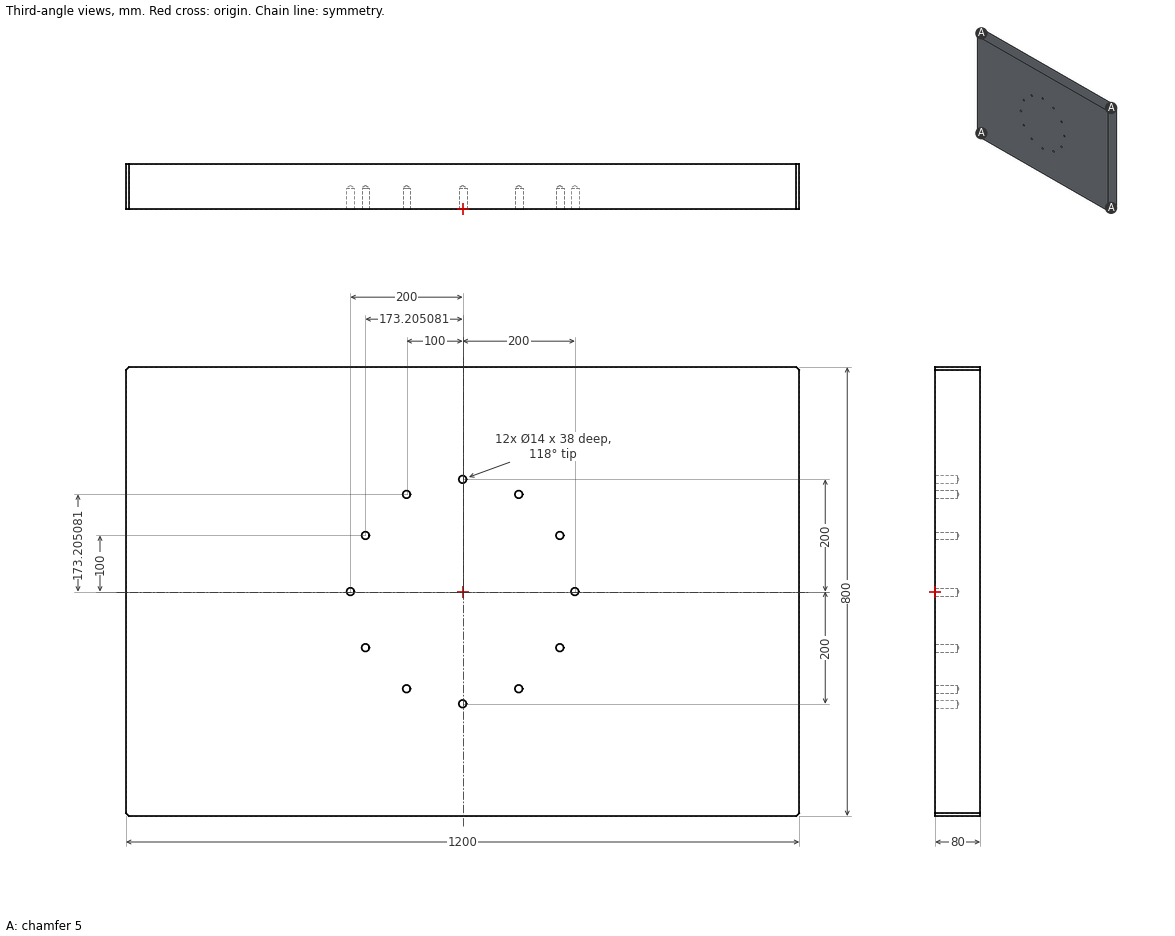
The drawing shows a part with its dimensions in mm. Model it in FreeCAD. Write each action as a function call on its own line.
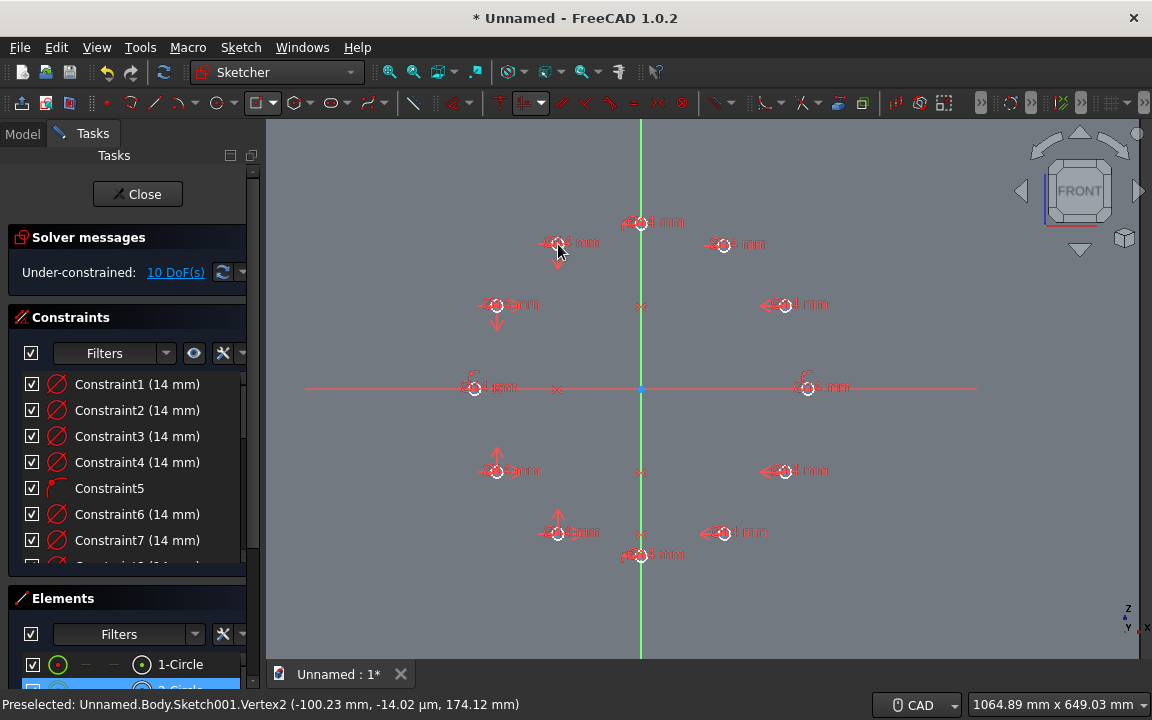
click(724, 246)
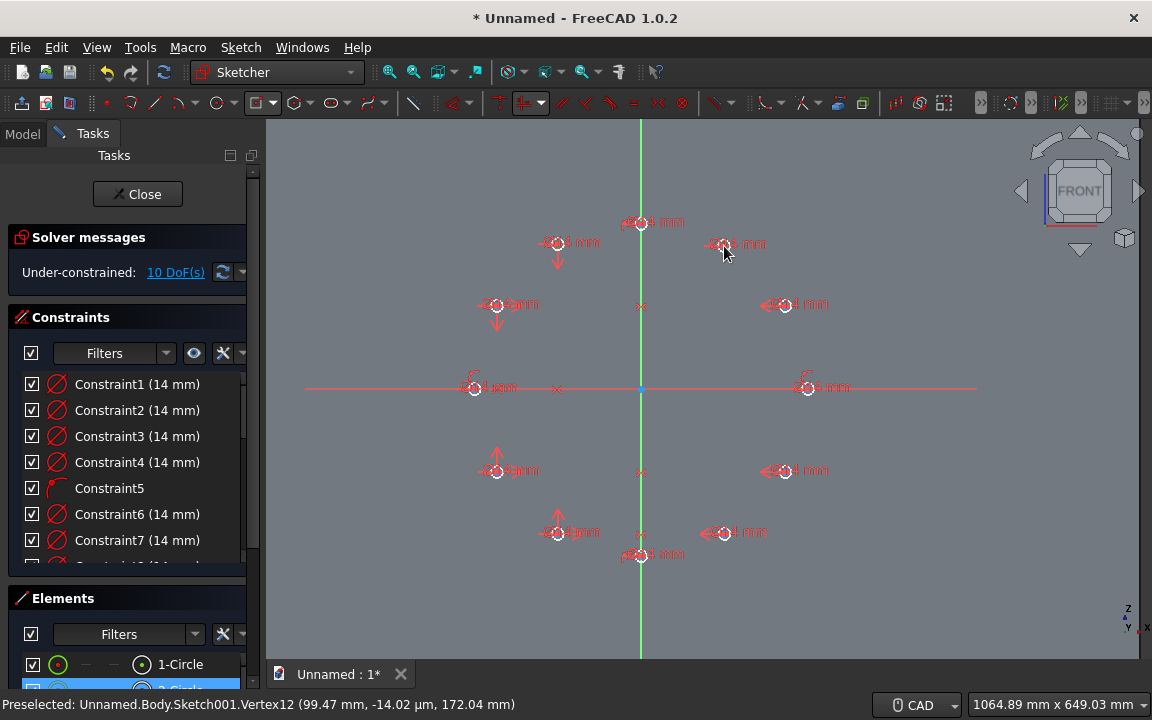
click(641, 596)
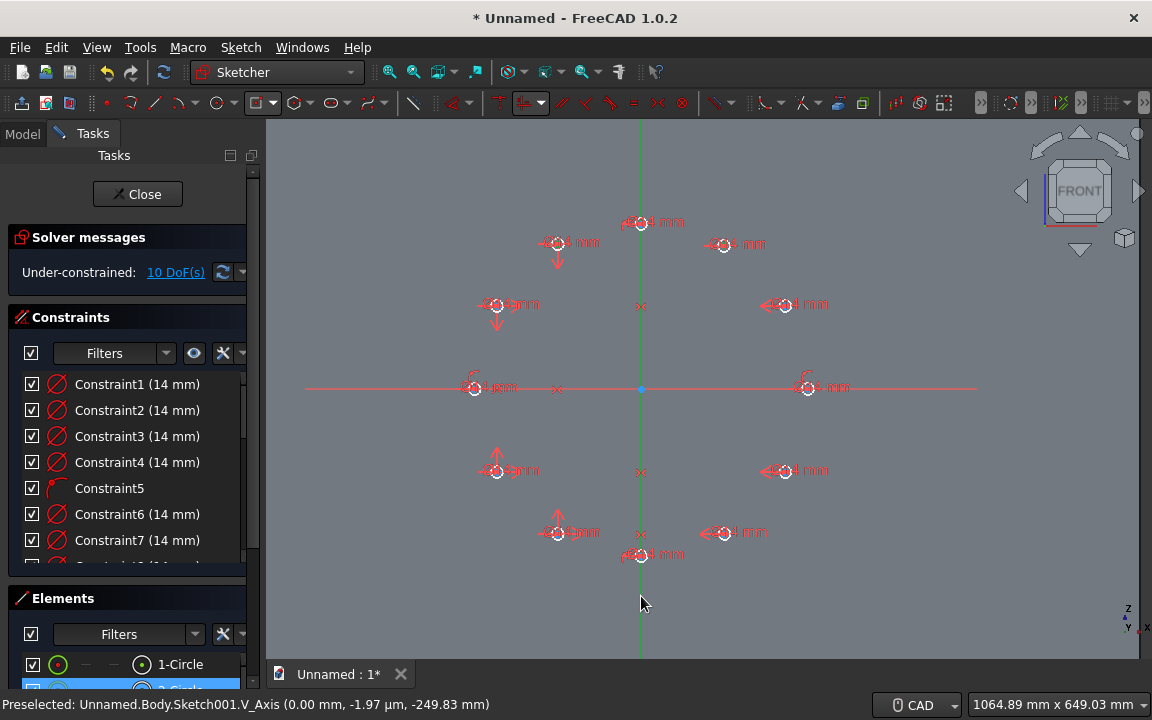
click(658, 104)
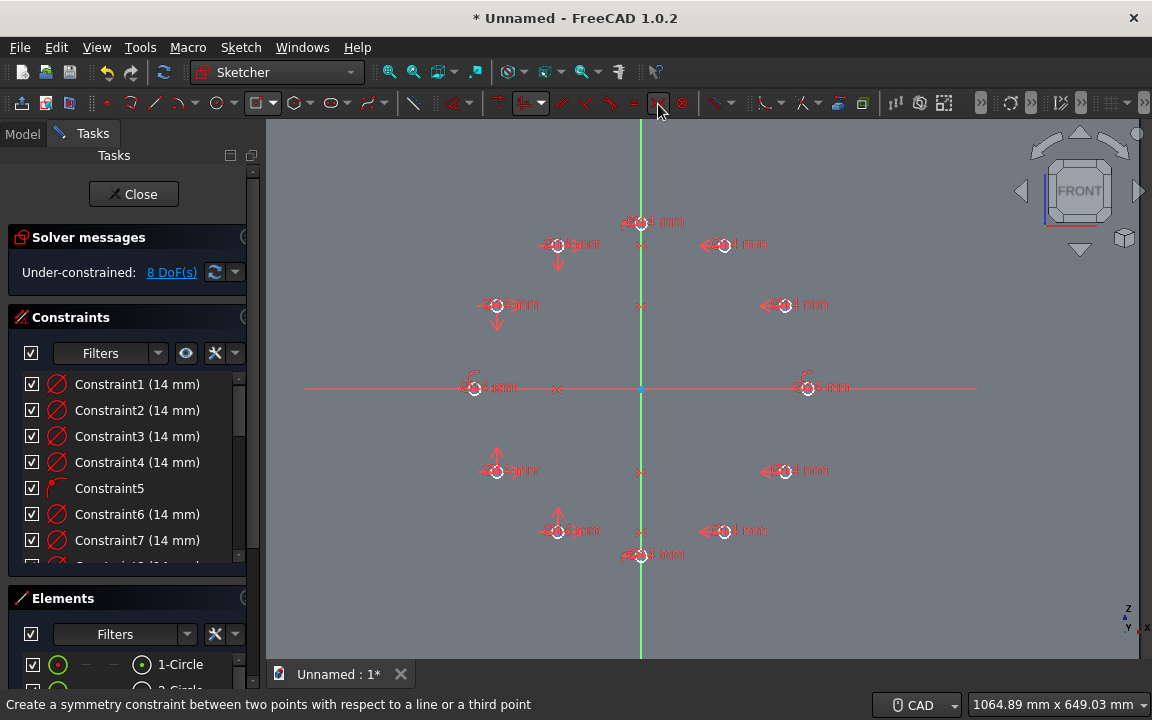
click(452, 104)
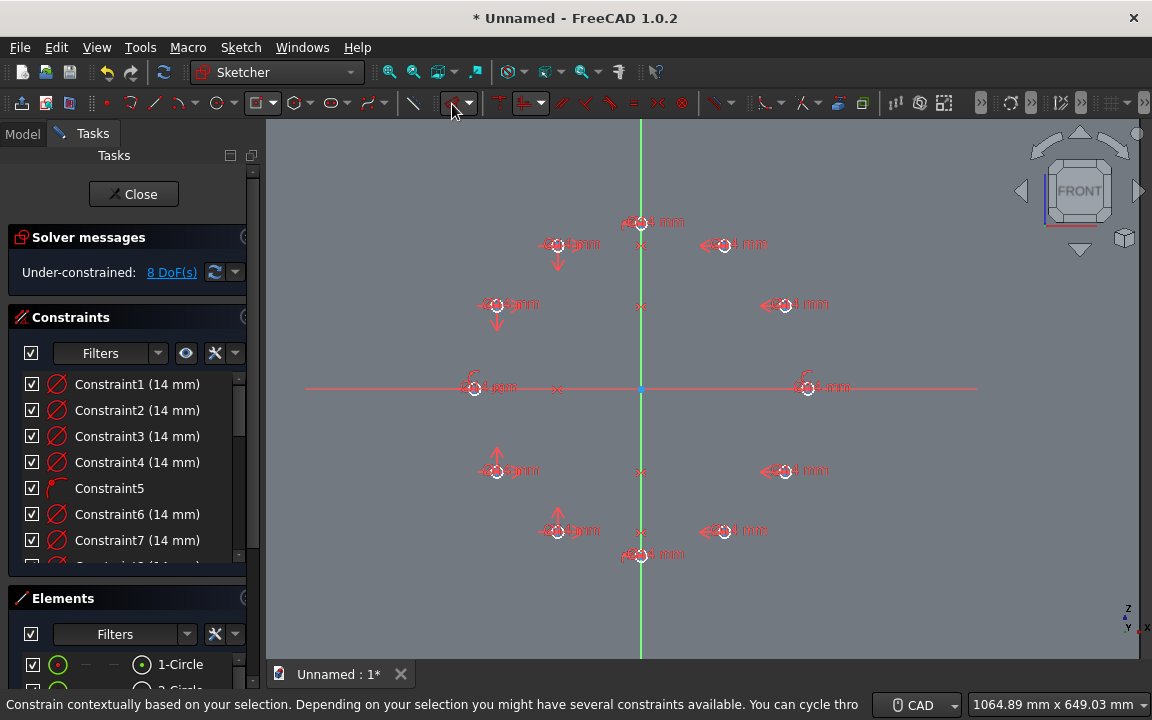
click(641, 224)
click(675, 307)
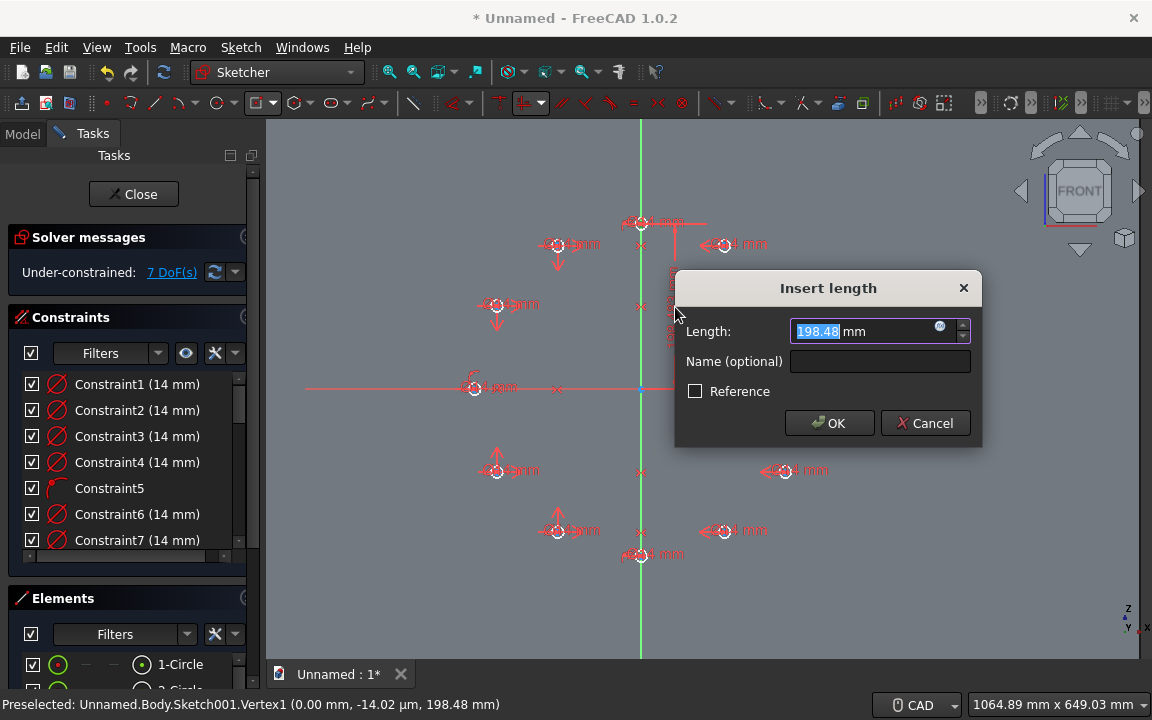
text(200)
key(Return)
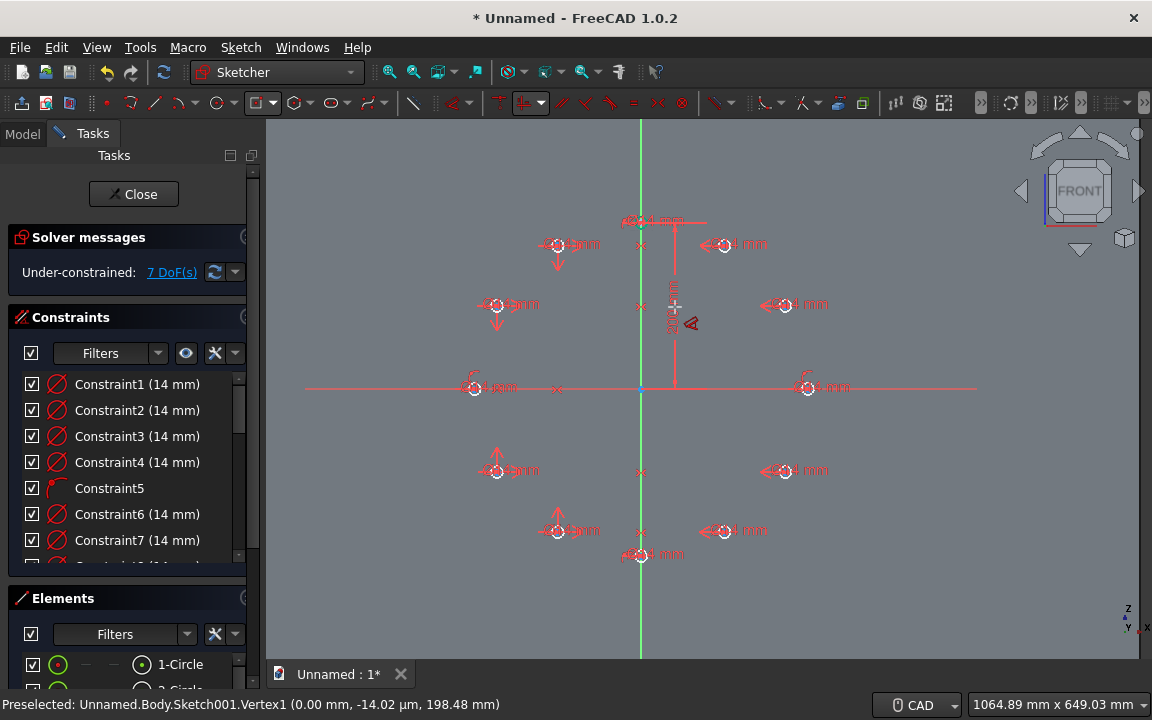
click(558, 246)
click(600, 212)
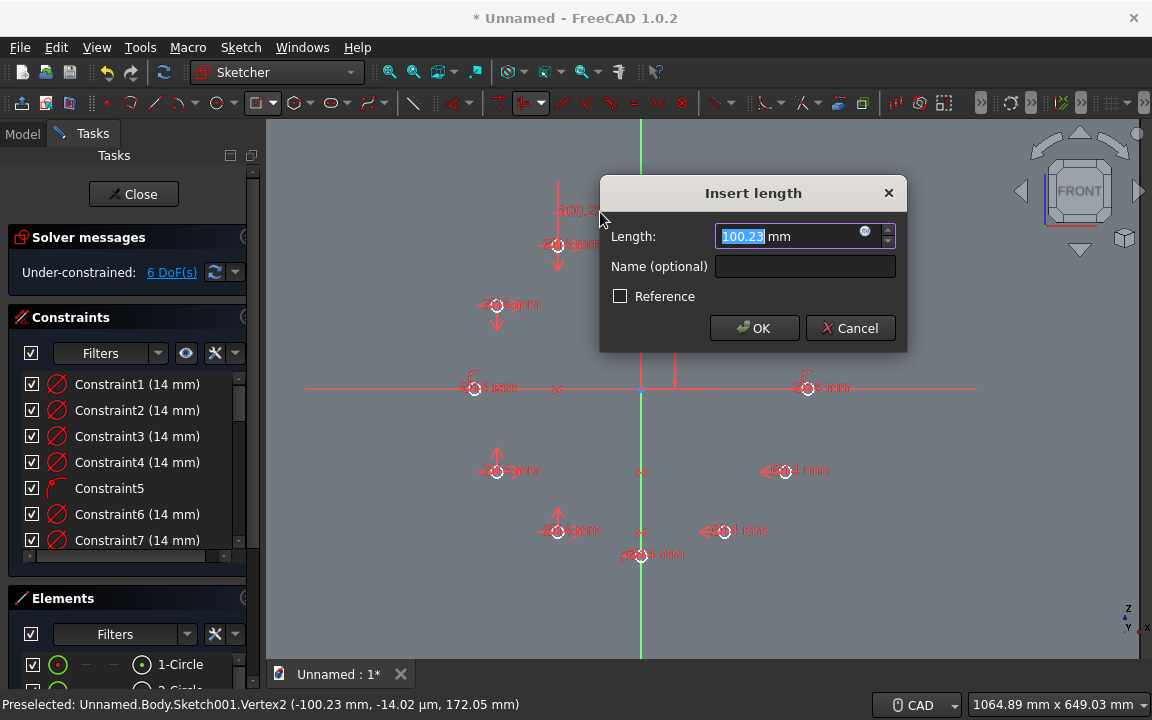
text(100)
key(Return)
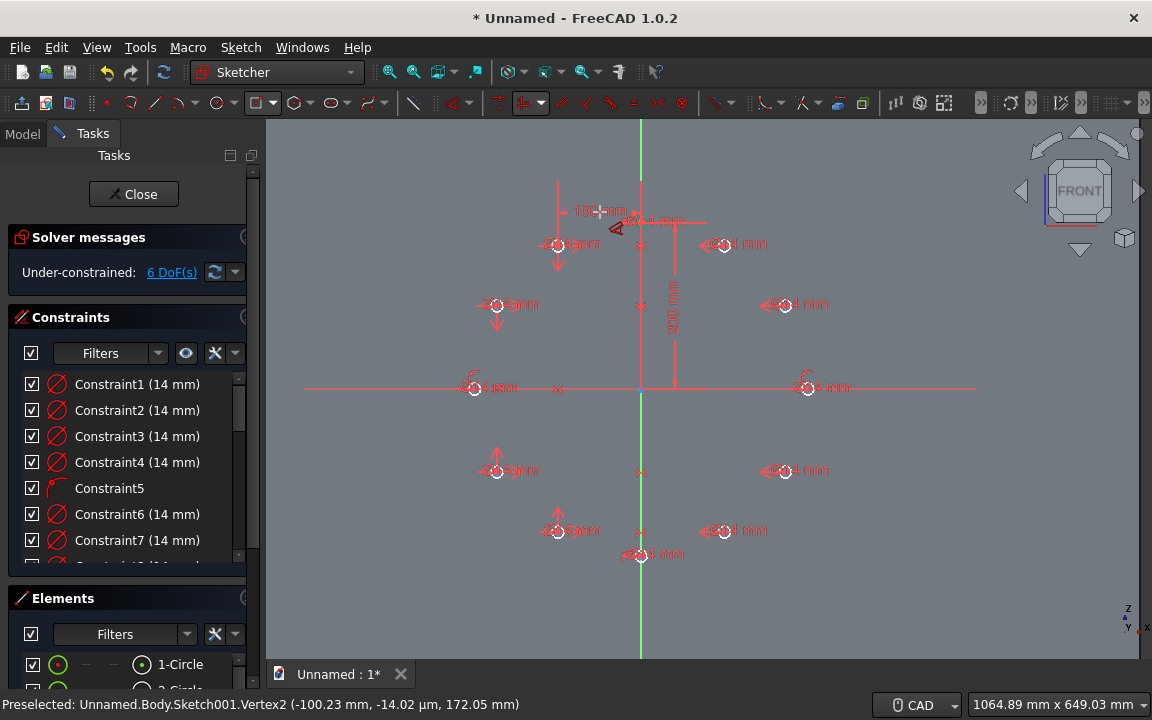
click(497, 306)
click(463, 348)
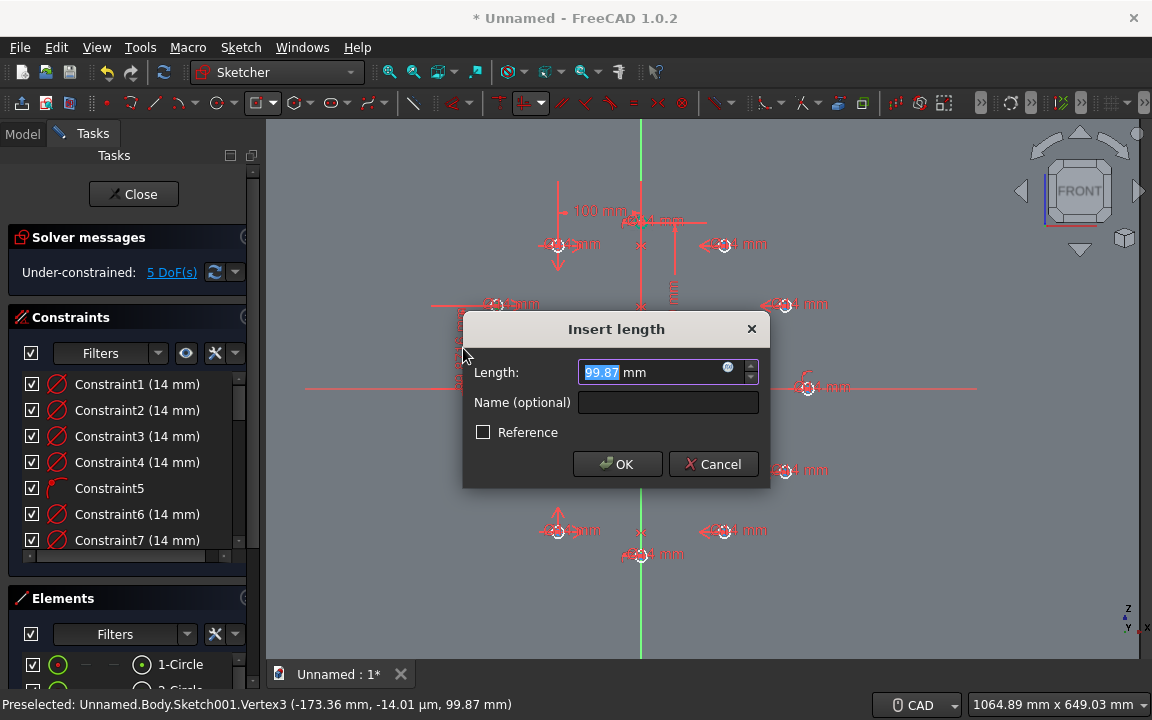
text(100)
key(Return)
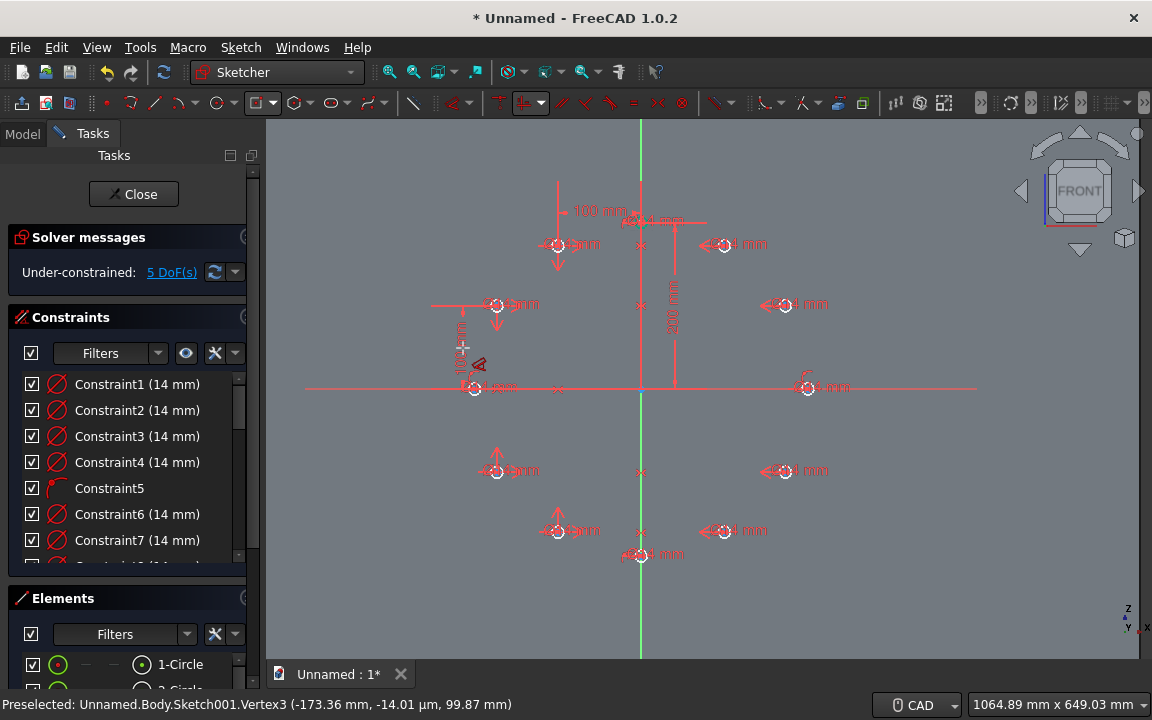
click(475, 389)
click(558, 423)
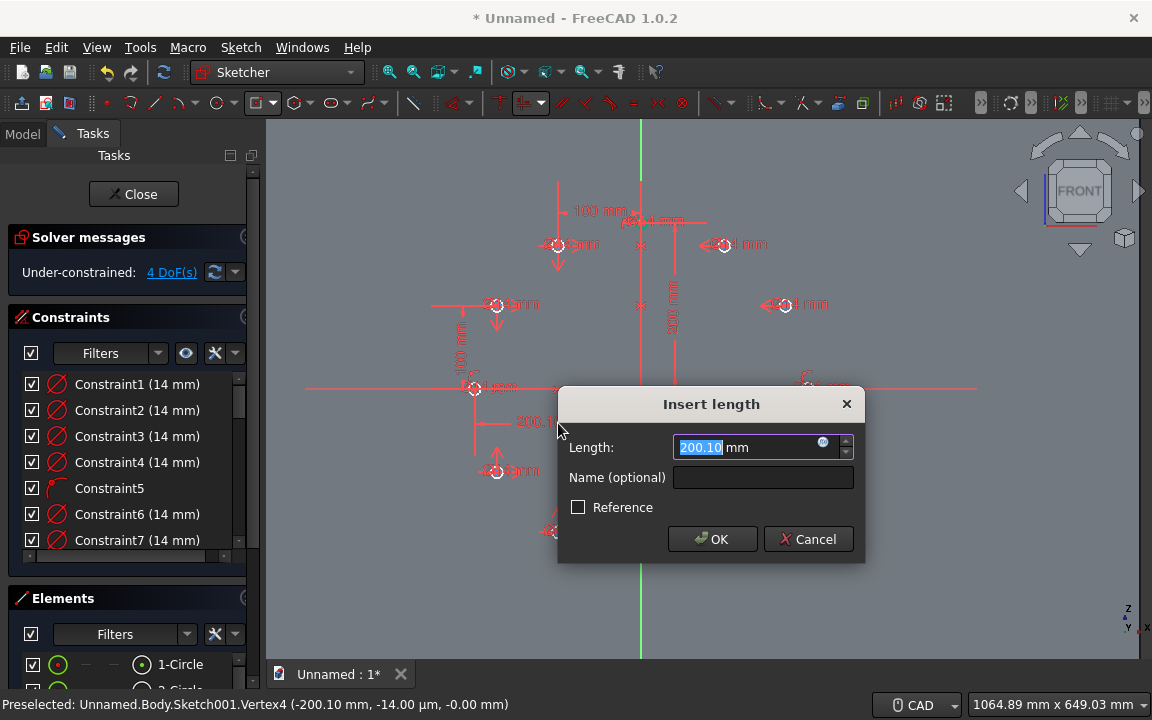
text(200)
key(Return)